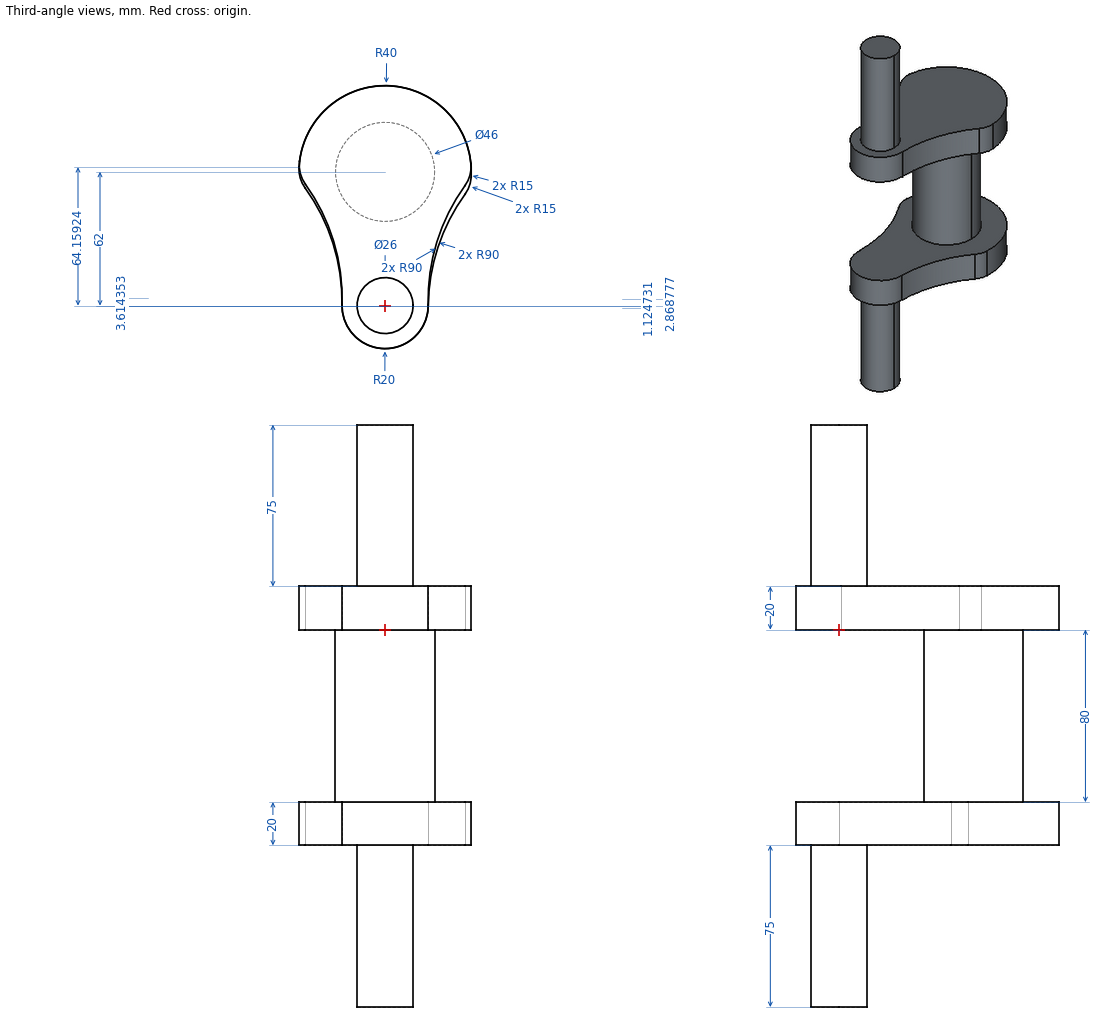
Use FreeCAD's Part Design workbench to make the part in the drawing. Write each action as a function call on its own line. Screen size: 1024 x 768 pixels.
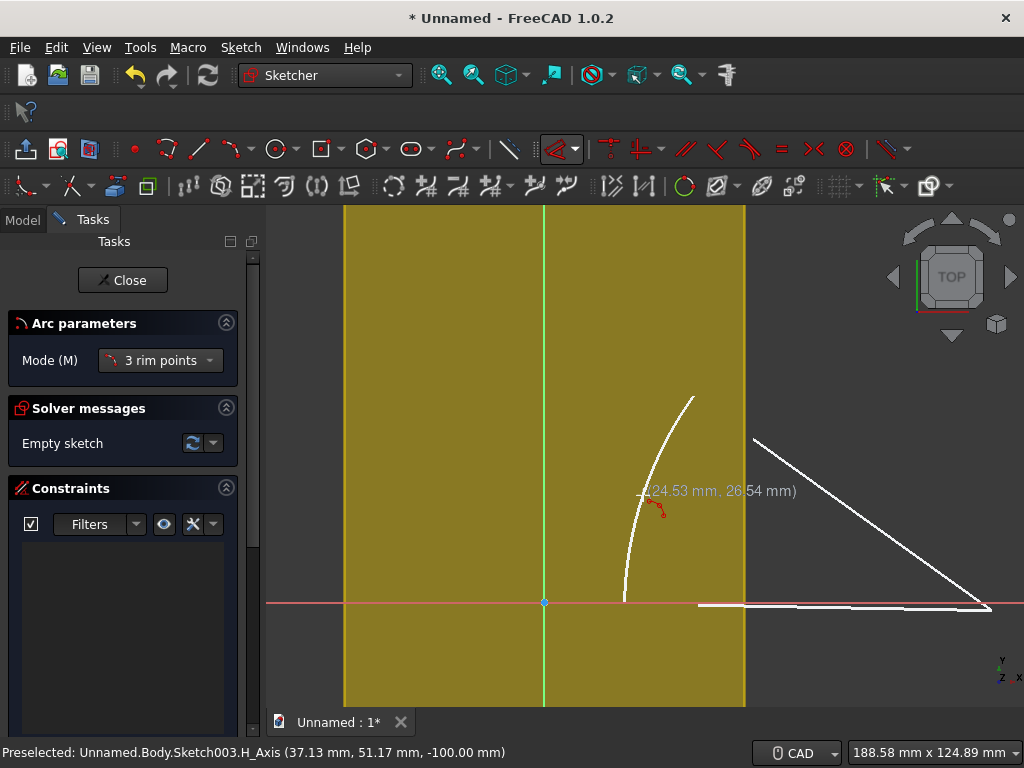
click(643, 494)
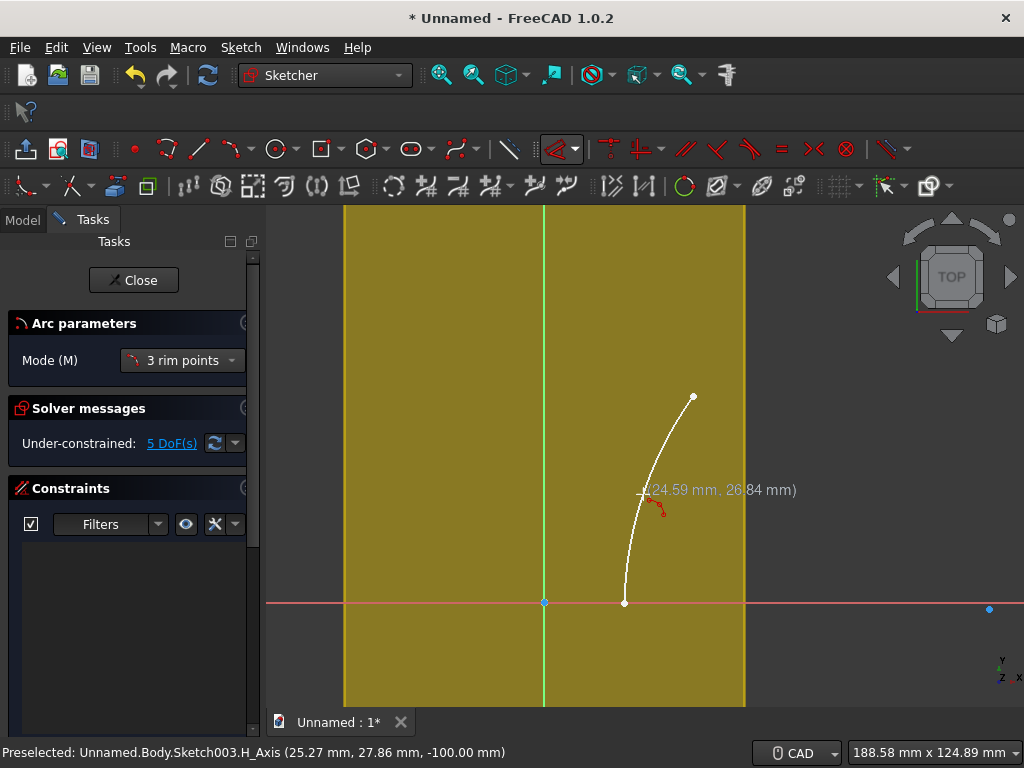
click(693, 396)
click(705, 364)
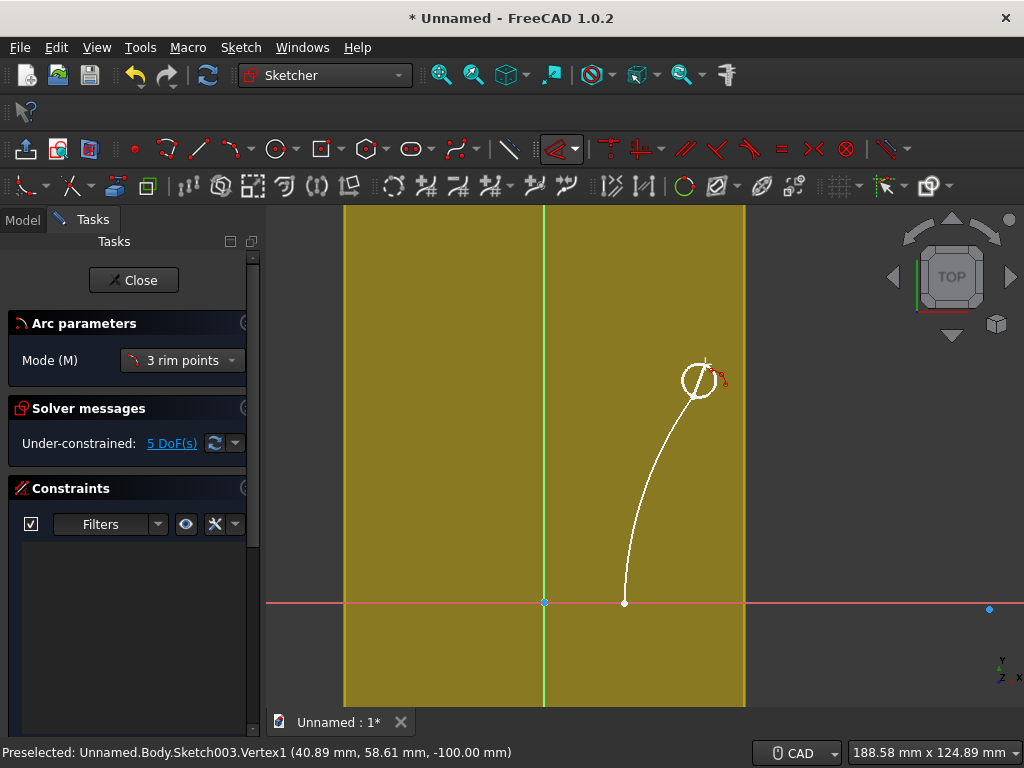
scroll(701, 380, up, 10)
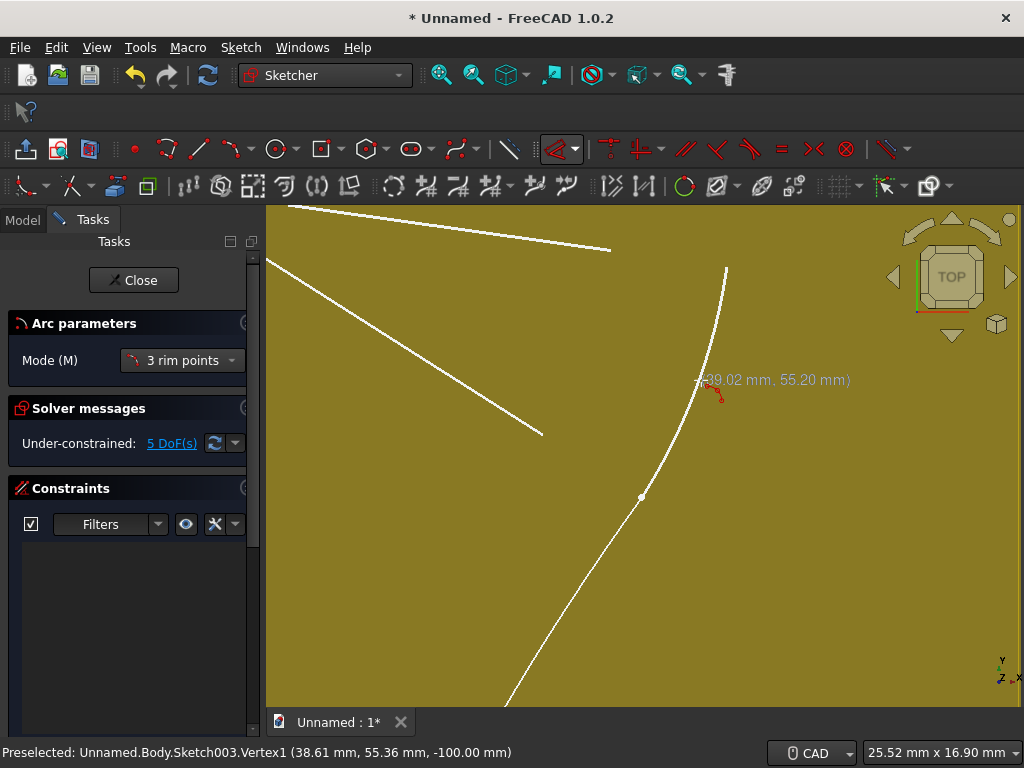
click(699, 379)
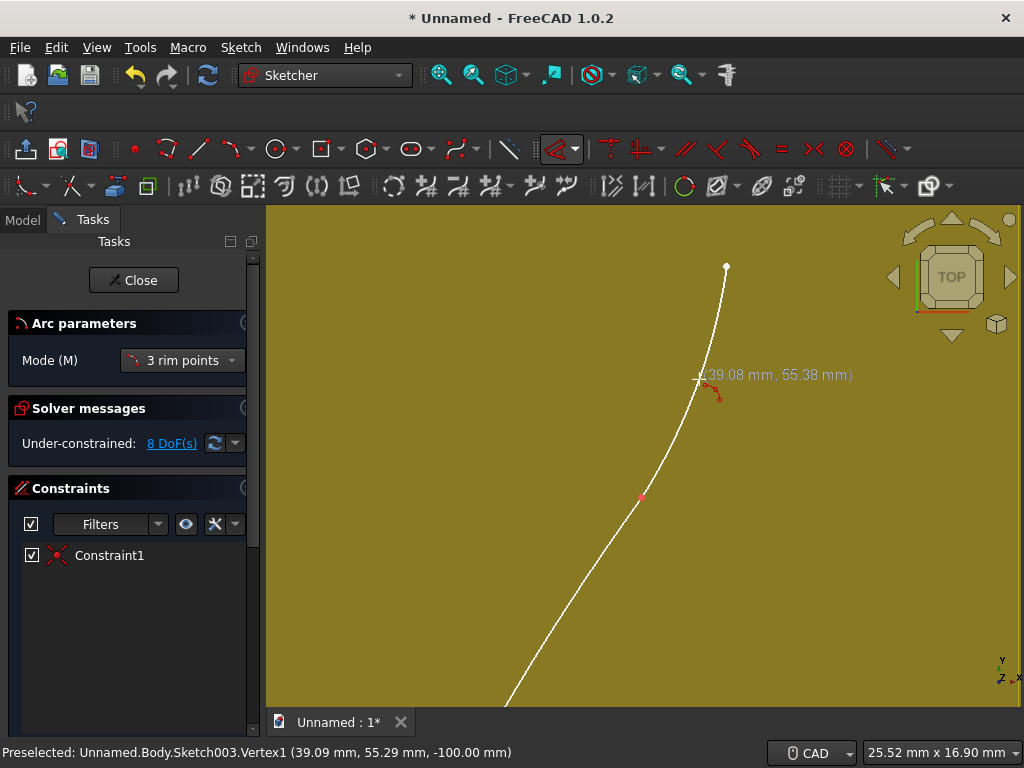
scroll(680, 421, down, 12)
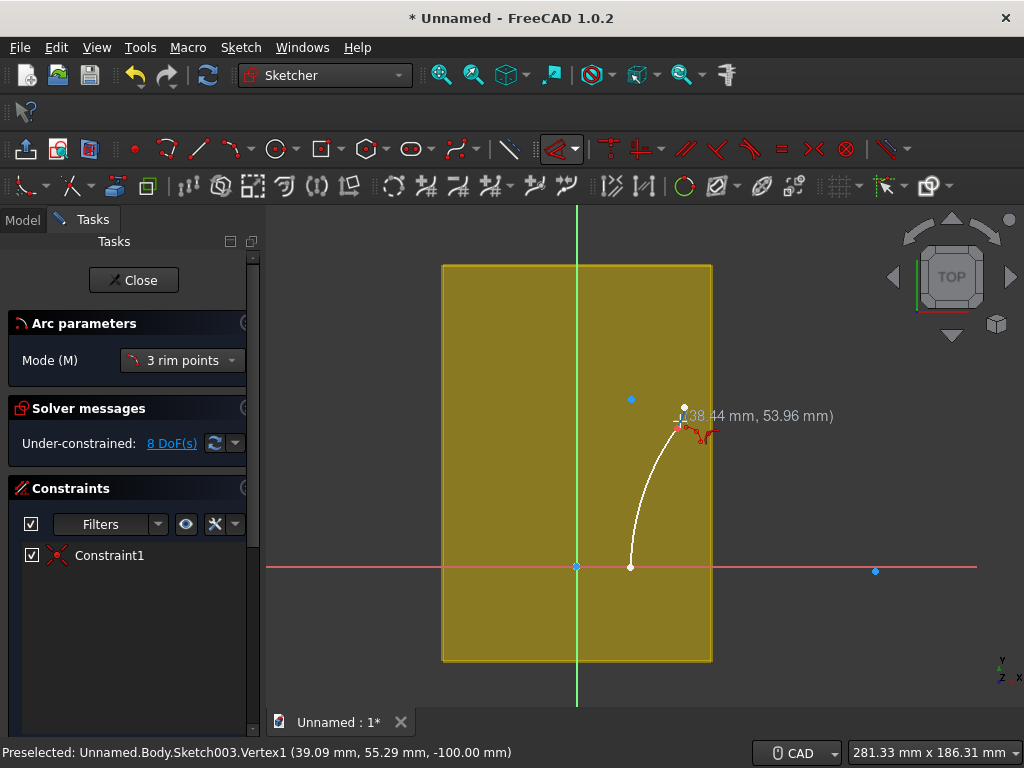
click(685, 407)
click(469, 394)
click(616, 299)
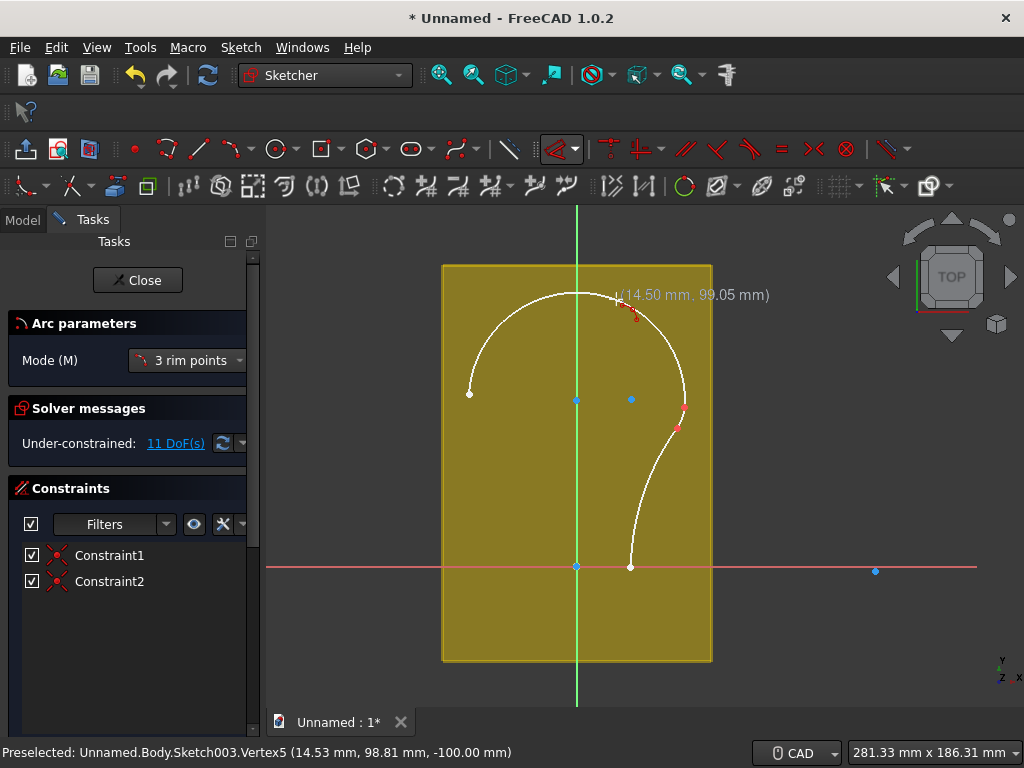
click(469, 395)
click(477, 420)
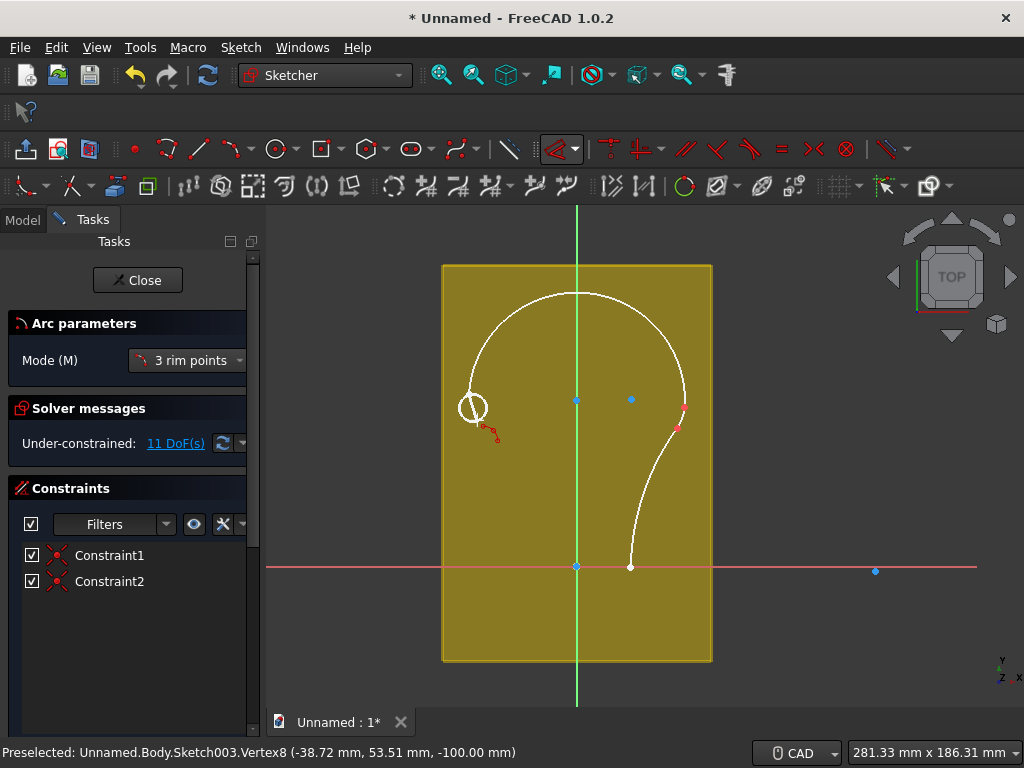
scroll(471, 408, up, 10)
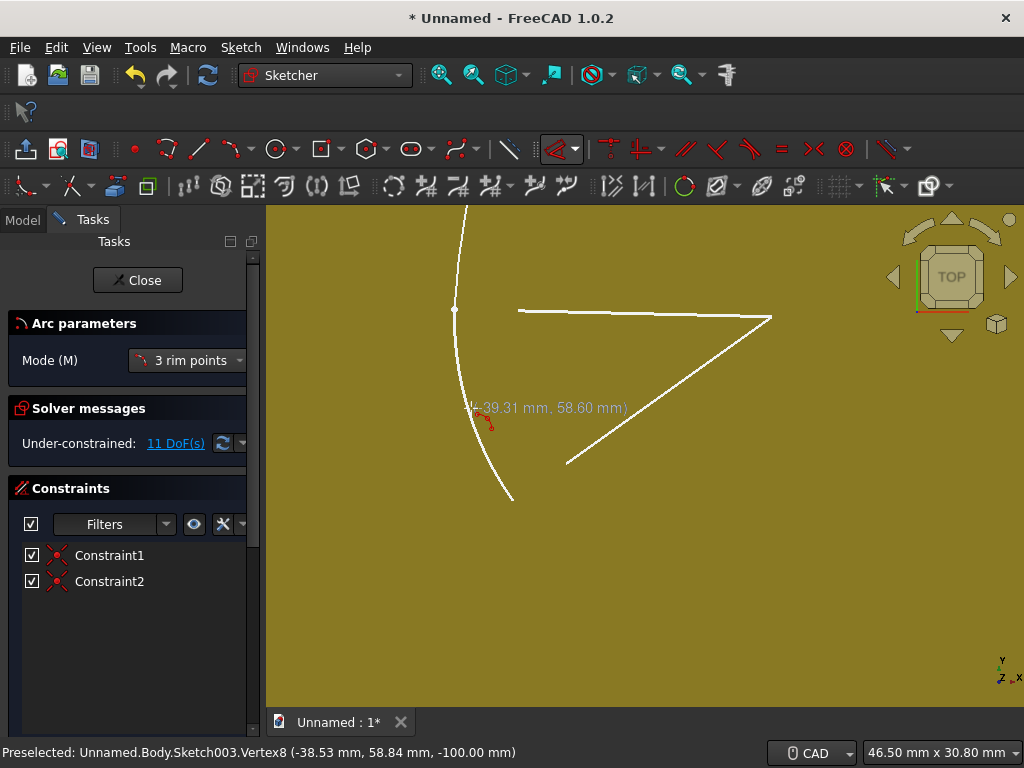
click(469, 403)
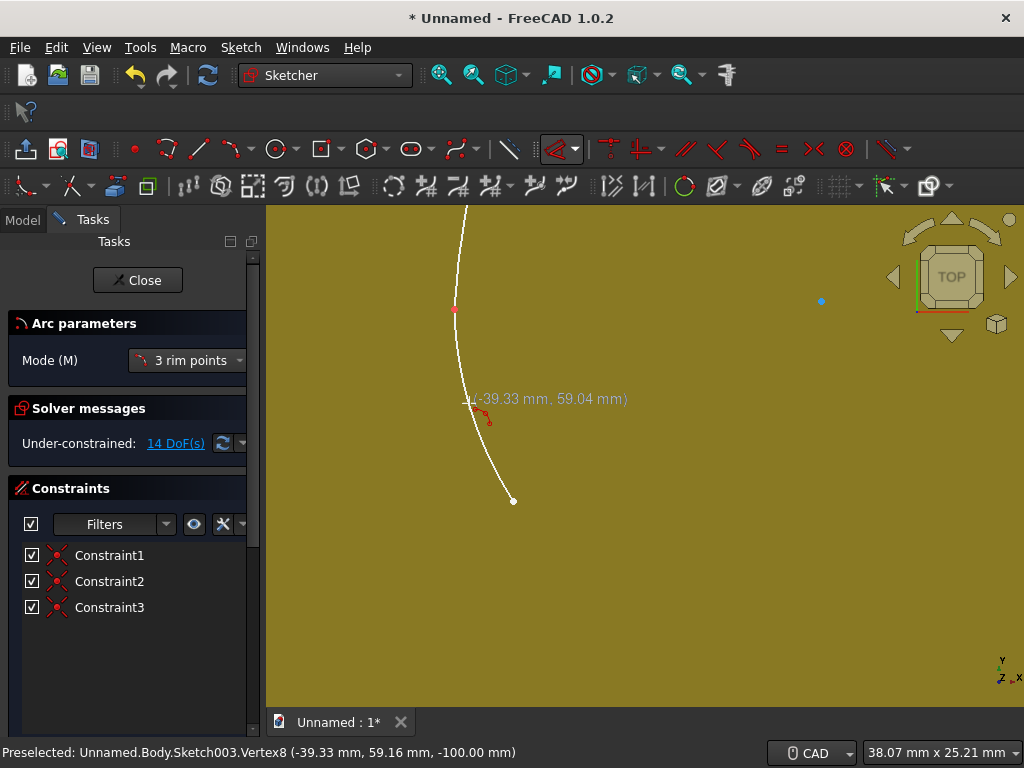
scroll(471, 408, down, 10)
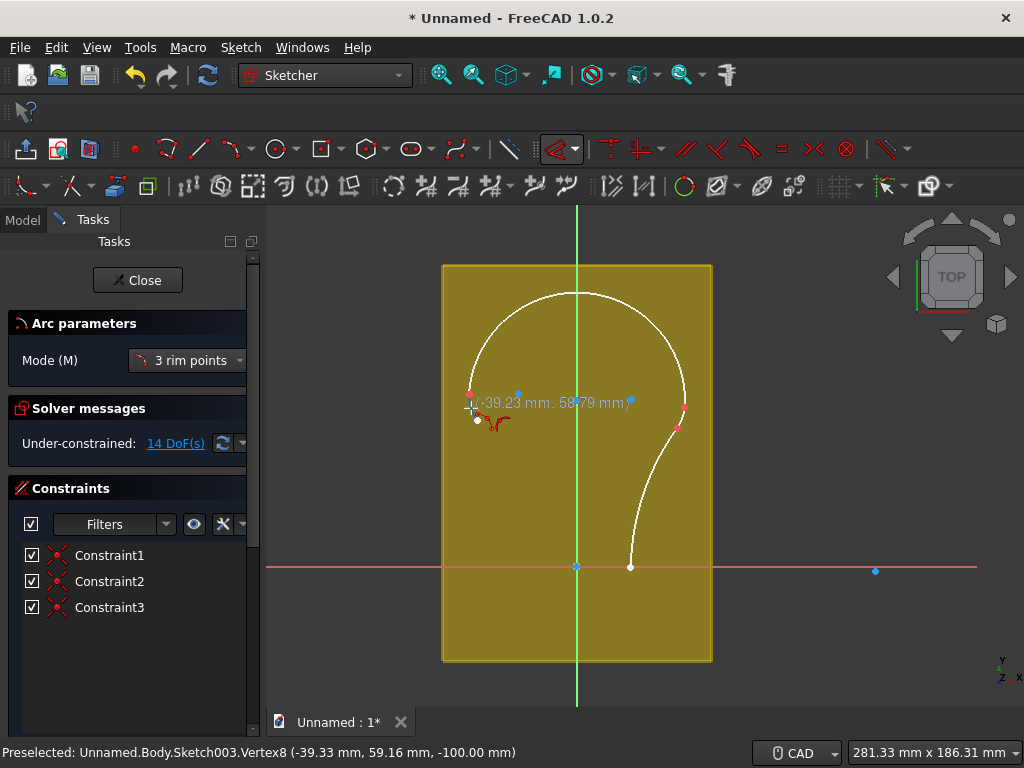
click(477, 421)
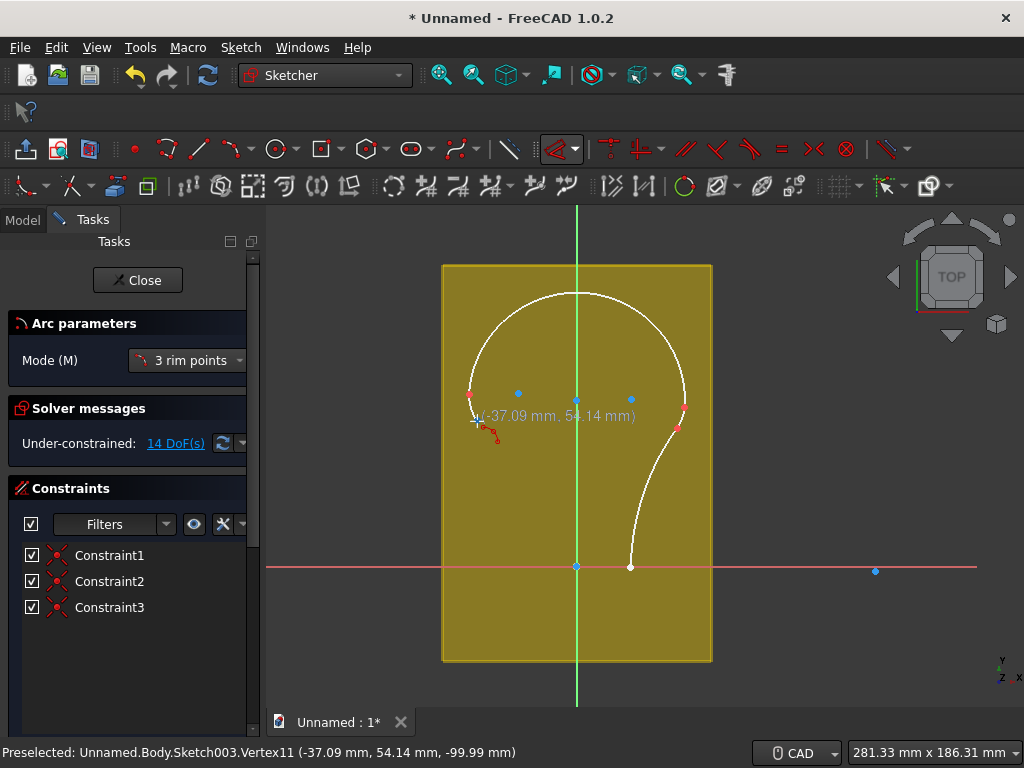
scroll(523, 566, up, 15)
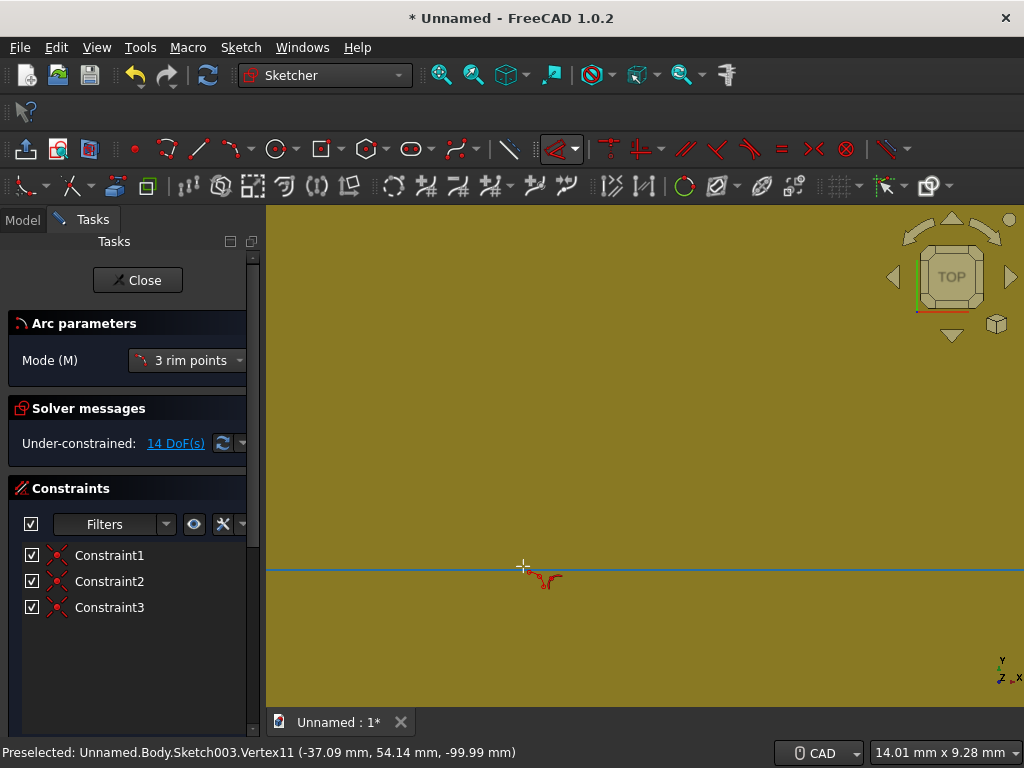
click(517, 553)